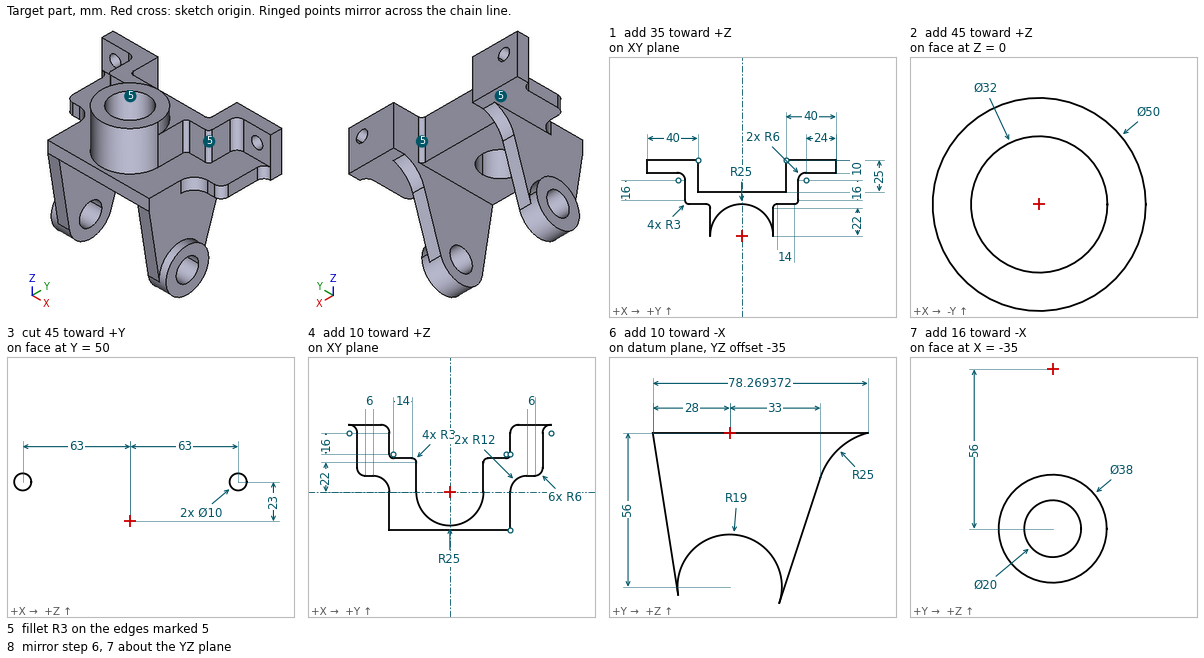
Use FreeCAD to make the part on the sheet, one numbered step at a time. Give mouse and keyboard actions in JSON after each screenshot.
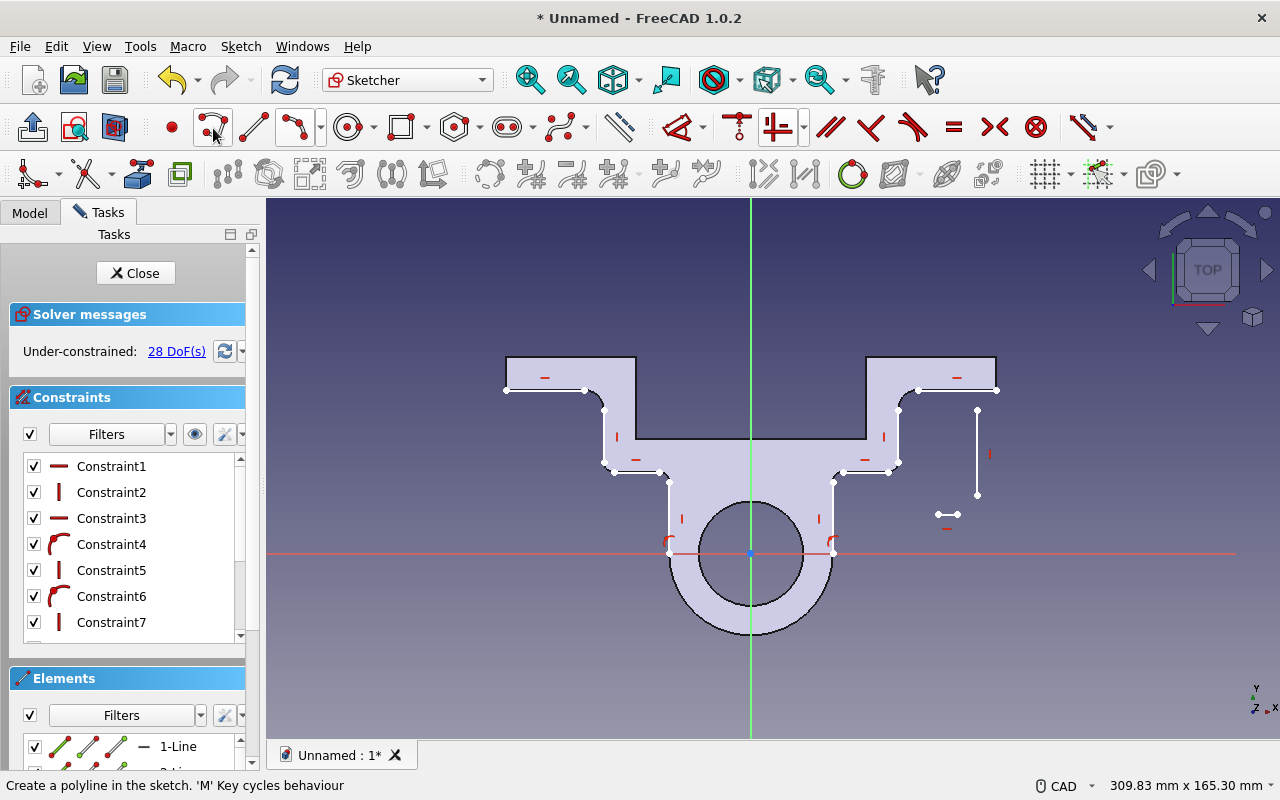
{"action": "left_click", "coordinate": [898, 554]}
{"action": "left_click", "coordinate": [898, 645]}
{"action": "left_click", "coordinate": [604, 645]}
{"action": "left_click", "coordinate": [604, 554]}
{"action": "right_click", "coordinate": [604, 554]}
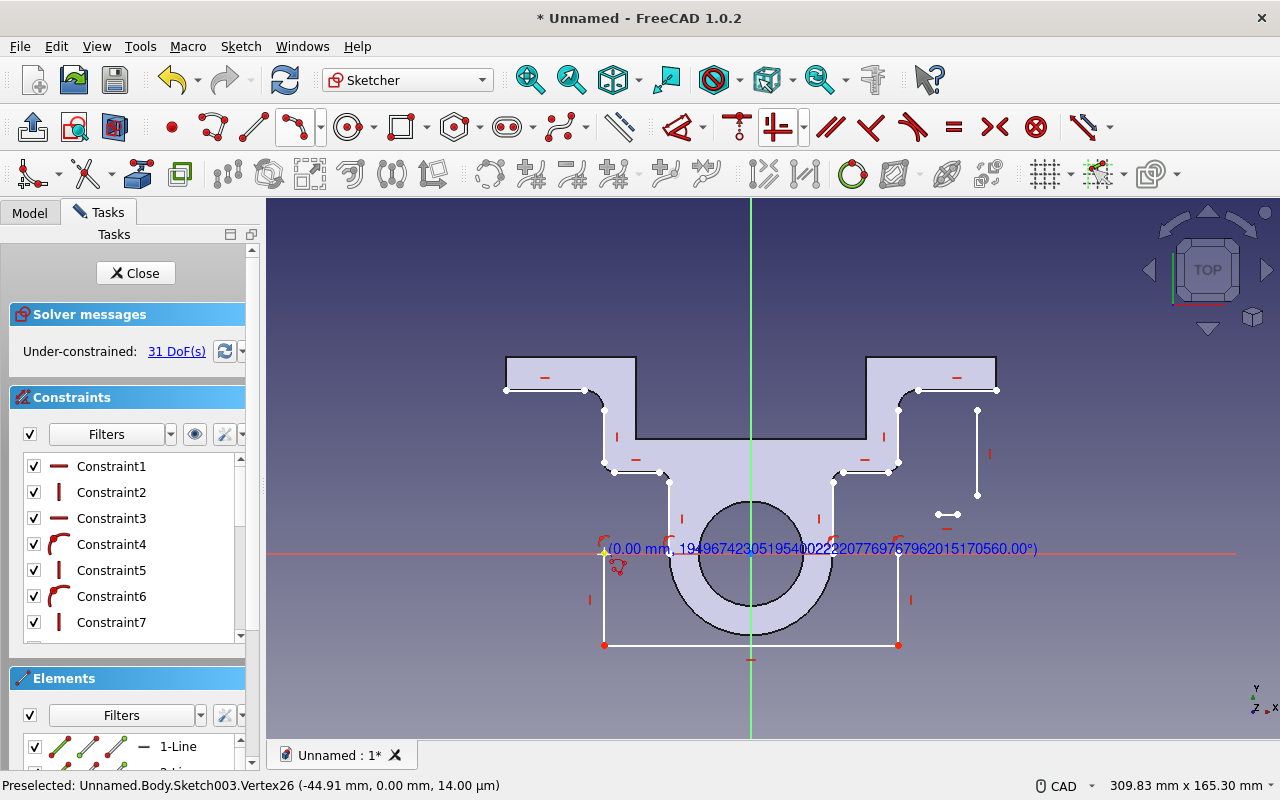
{"action": "left_click", "coordinate": [254, 128]}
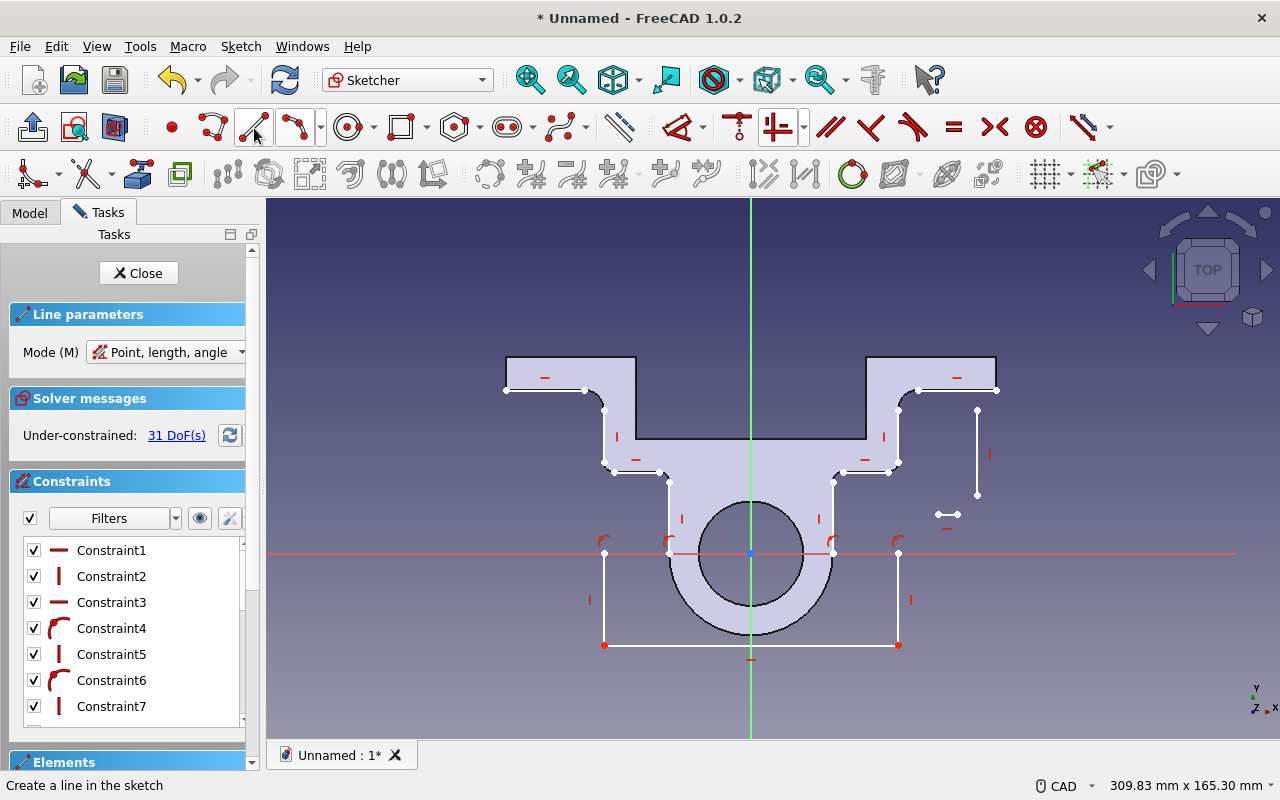
{"action": "left_click", "coordinate": [564, 514]}
{"action": "left_click", "coordinate": [545, 514]}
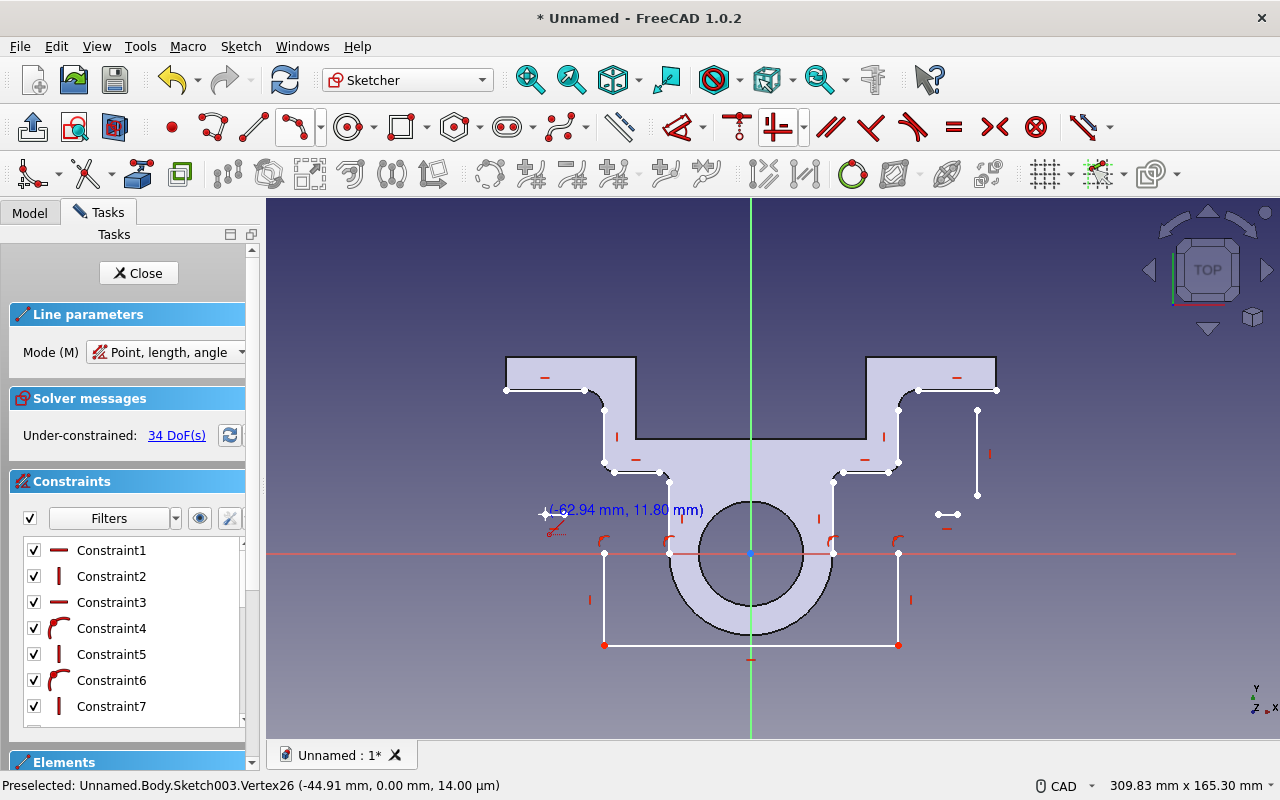
{"action": "left_click", "coordinate": [525, 495]}
{"action": "left_click", "coordinate": [525, 410]}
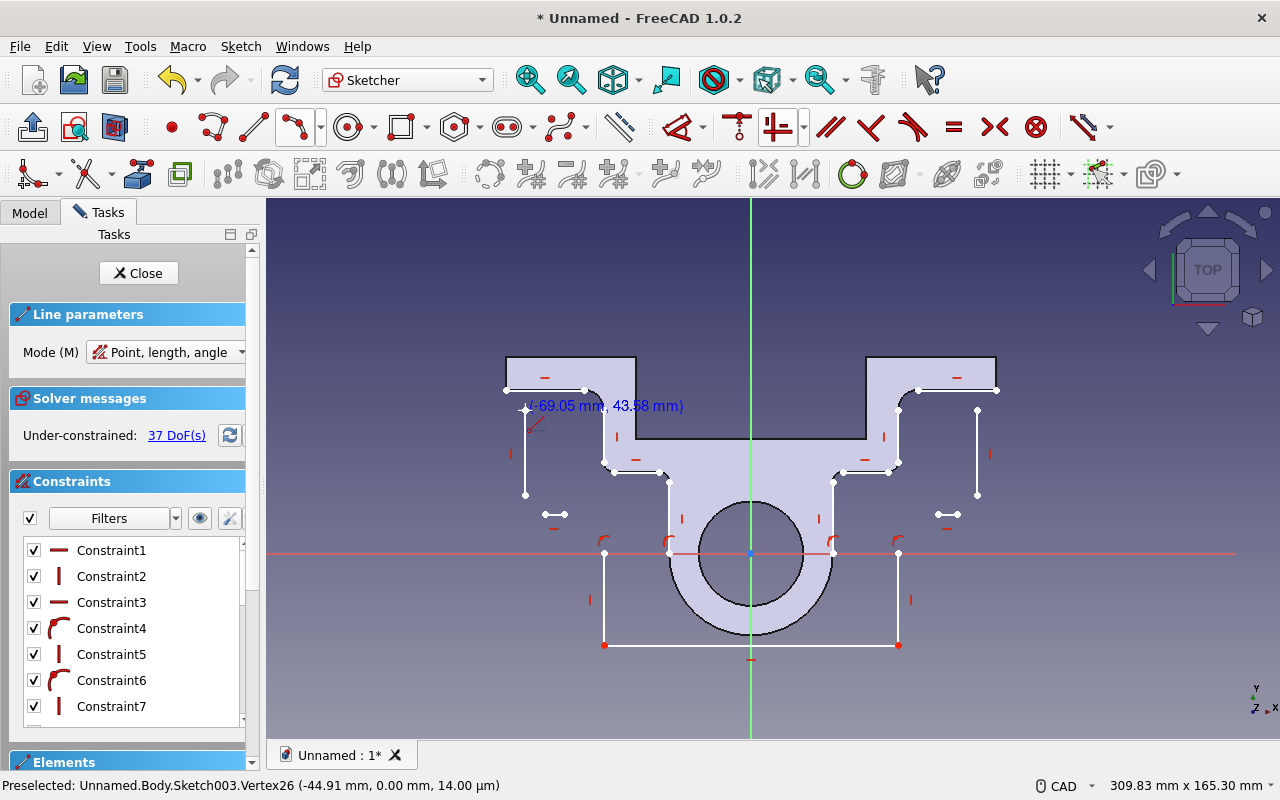
{"action": "left_click", "coordinate": [294, 128]}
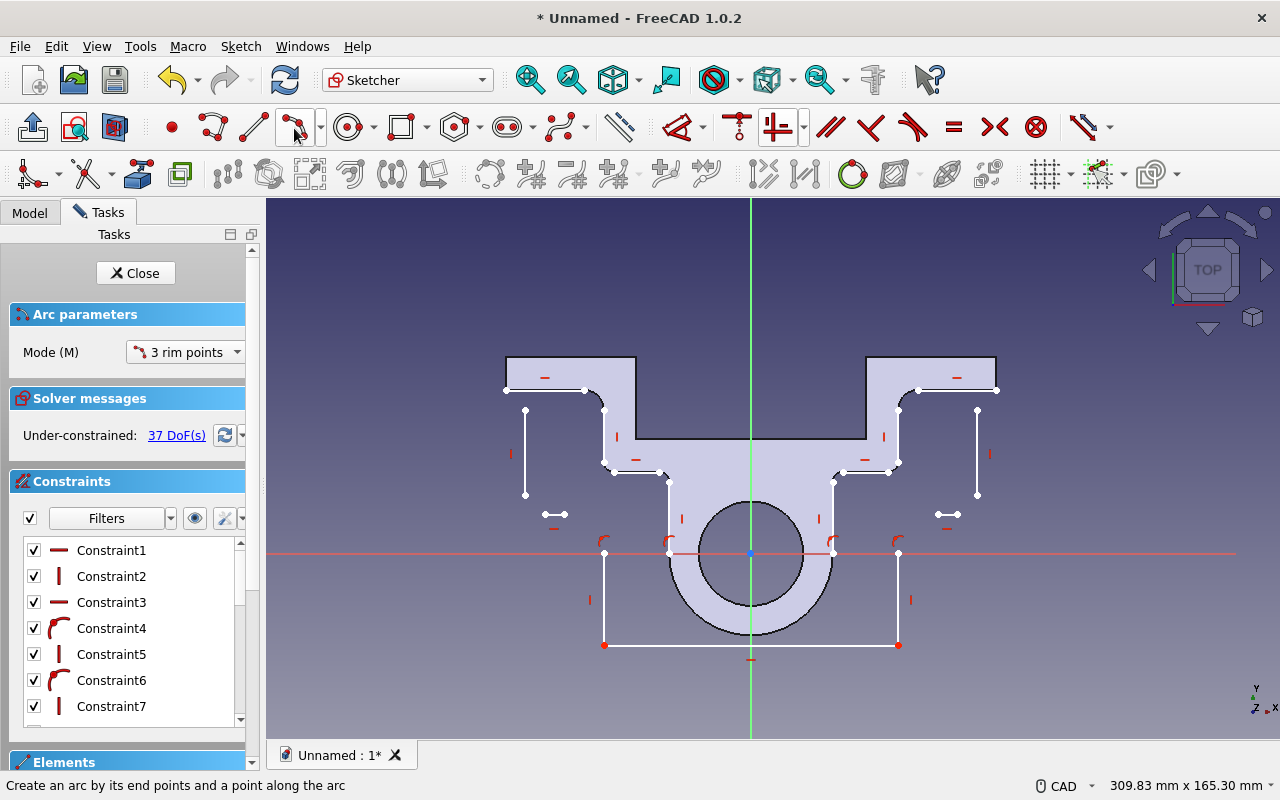
{"action": "left_click", "coordinate": [584, 391]}
{"action": "left_click", "coordinate": [604, 411]}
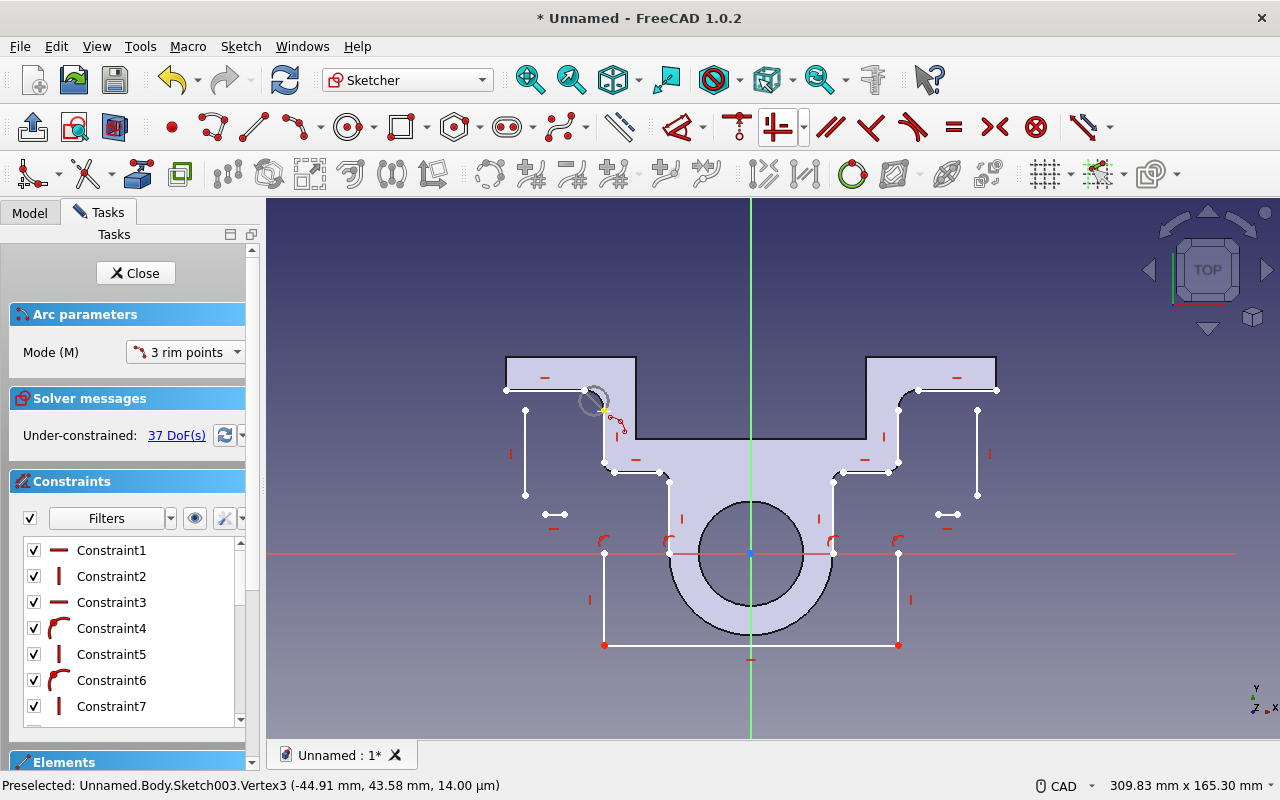
{"action": "scroll", "coordinate": [598, 396], "scroll_direction": "up", "scroll_amount": 6}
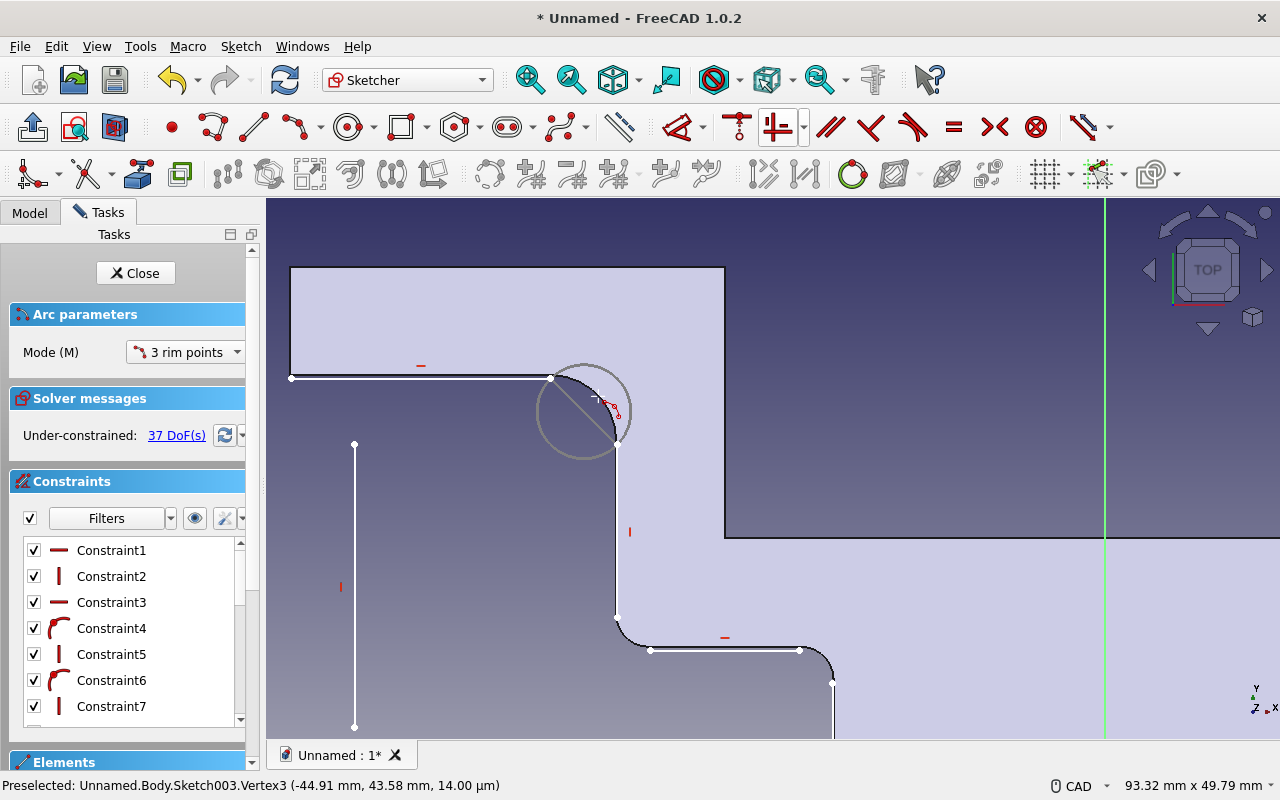
{"action": "left_click", "coordinate": [597, 394]}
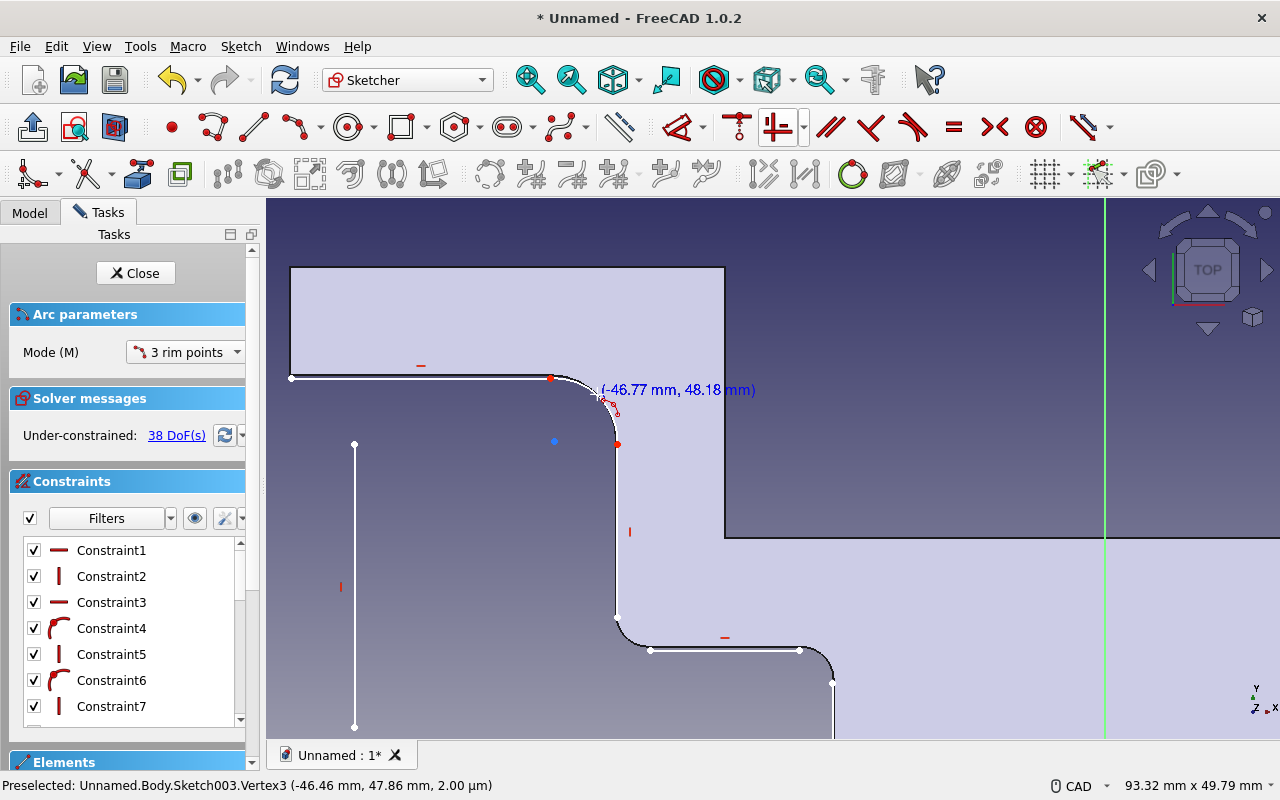
{"action": "left_click", "coordinate": [617, 618]}
{"action": "left_click", "coordinate": [650, 651]}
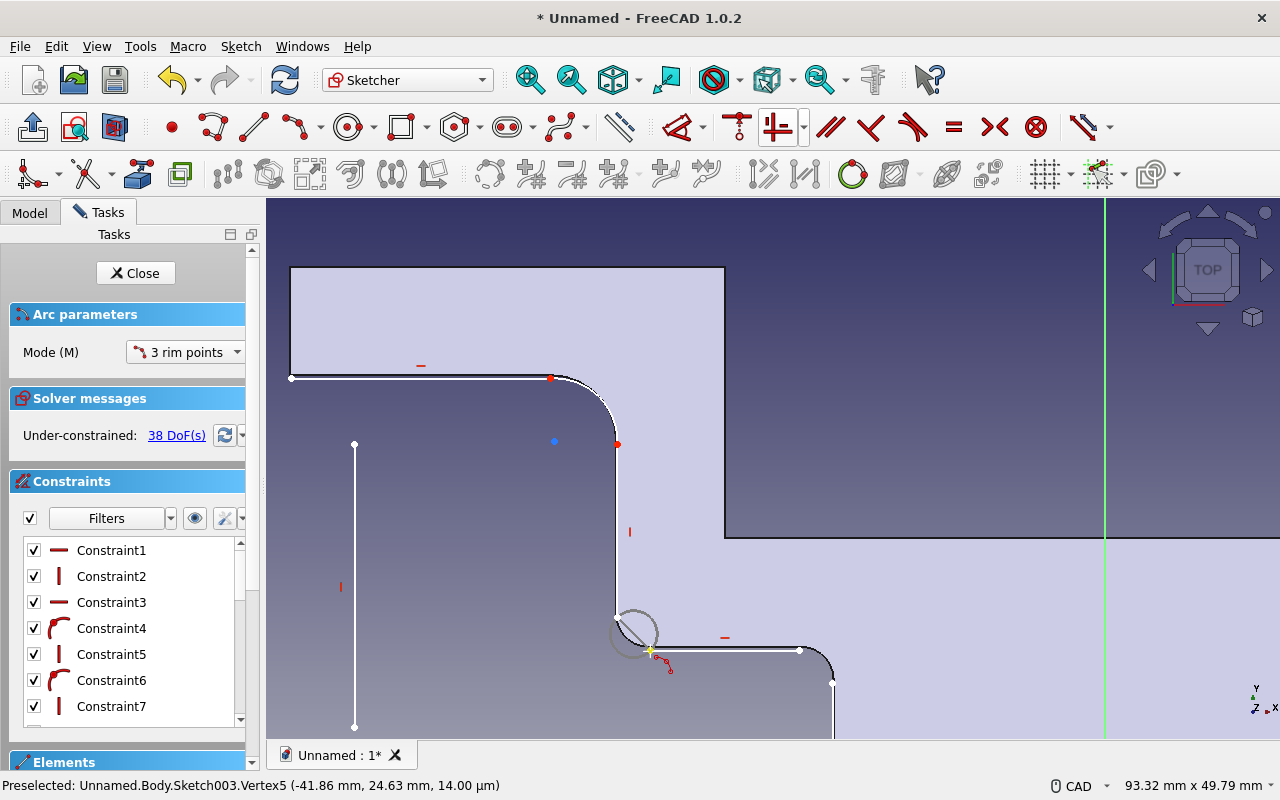
{"action": "scroll", "coordinate": [626, 637], "scroll_direction": "up", "scroll_amount": 3}